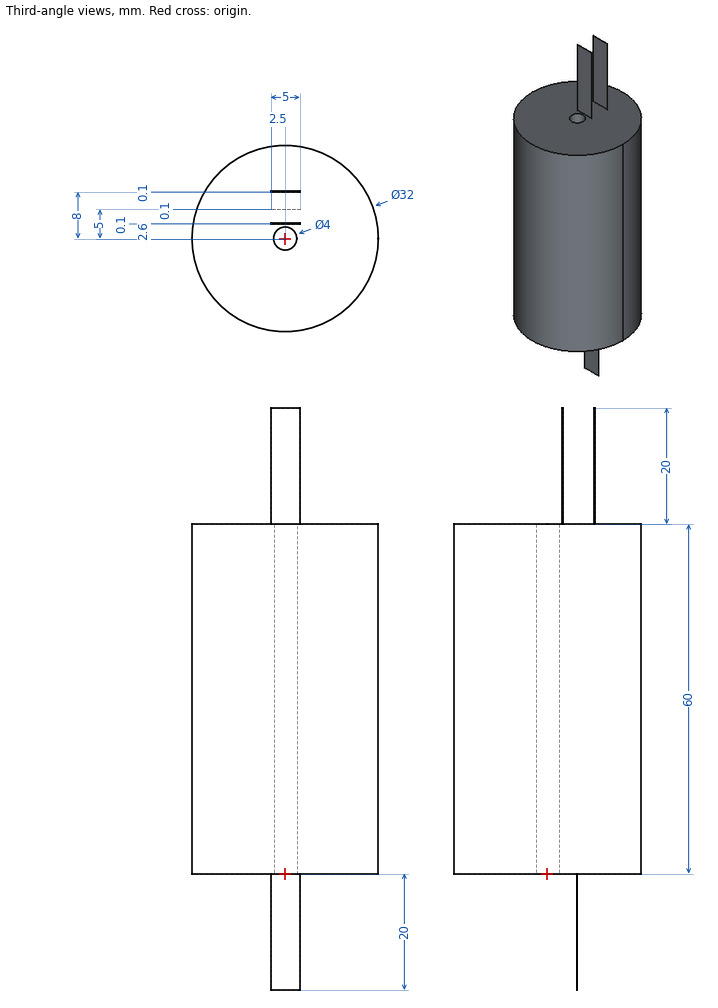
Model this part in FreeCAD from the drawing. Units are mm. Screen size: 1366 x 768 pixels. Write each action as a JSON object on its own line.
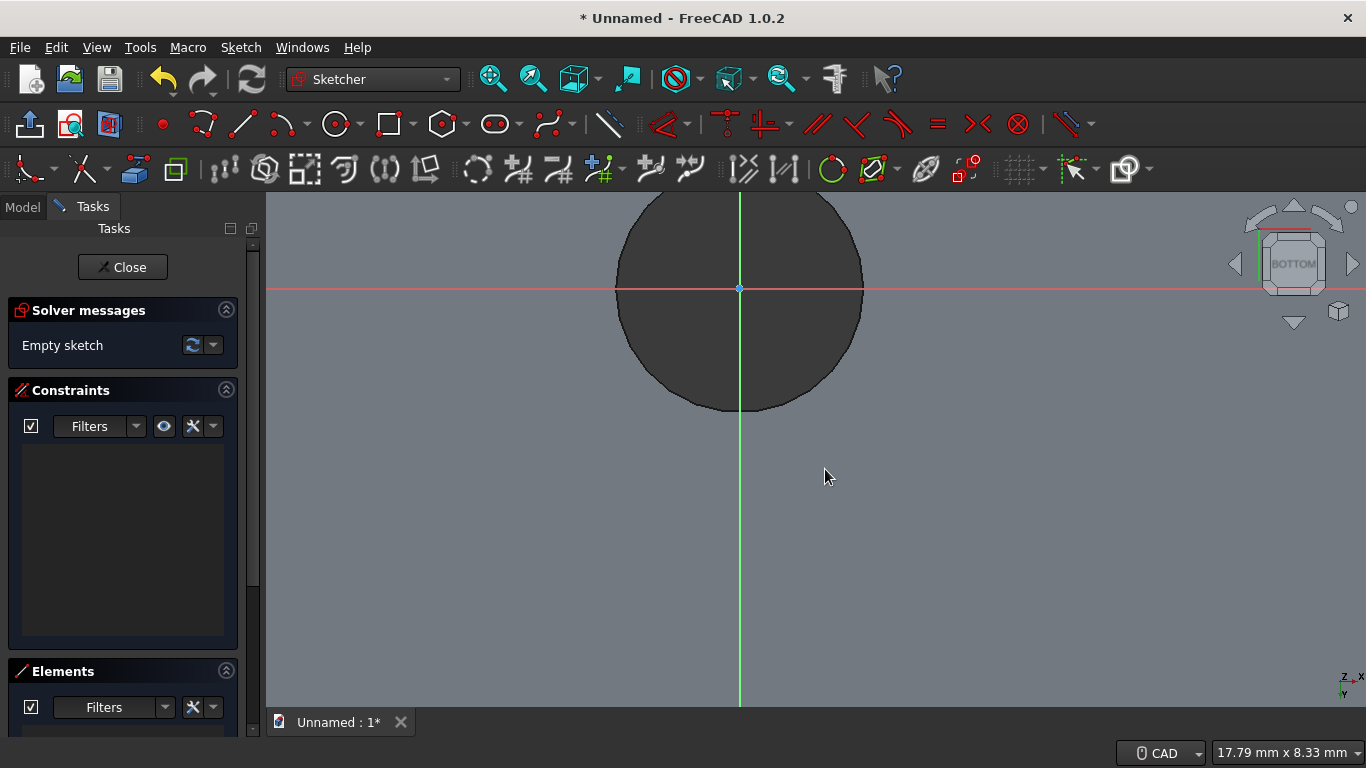
{"action": "left_click", "coordinate": [390, 124]}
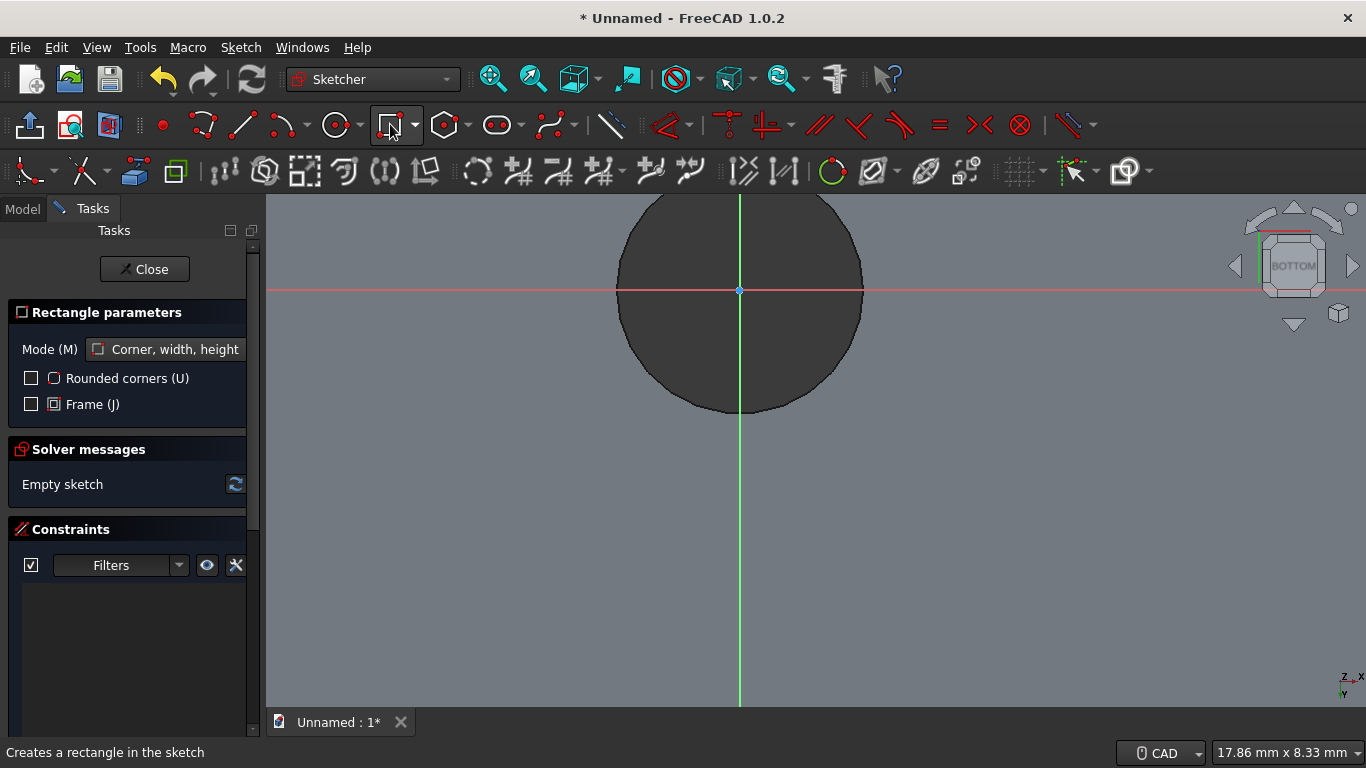
{"action": "scroll", "coordinate": [586, 598], "scroll_direction": "up", "scroll_amount": 5}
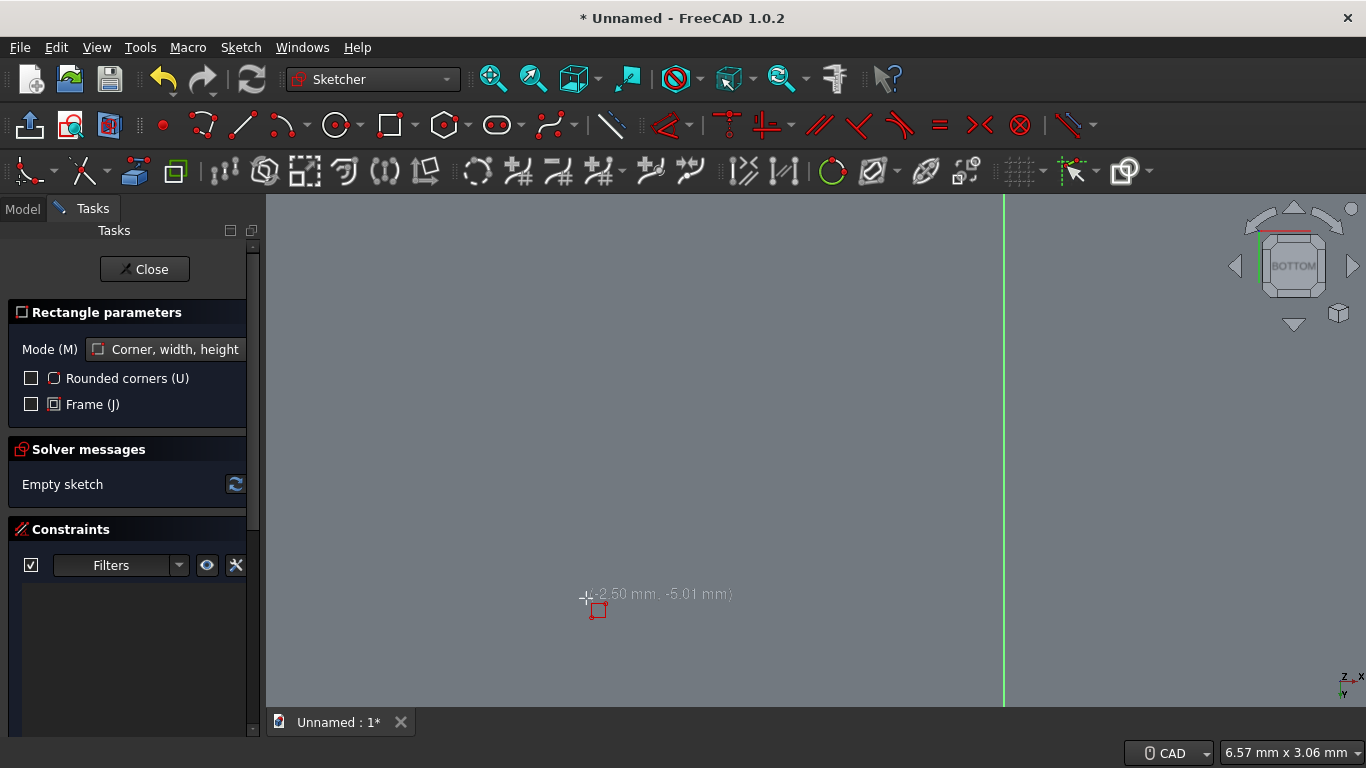
{"action": "left_click", "coordinate": [585, 598]}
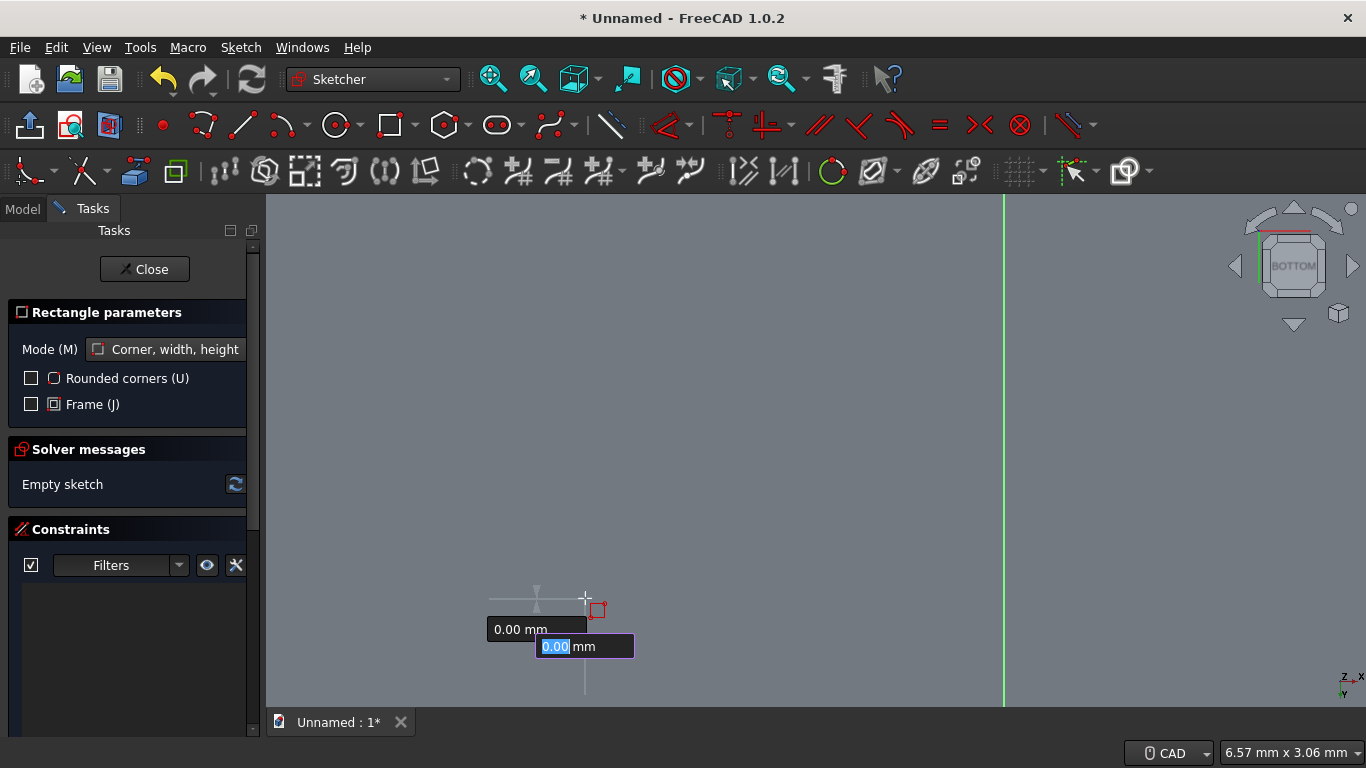
{"action": "scroll", "coordinate": [598, 604], "scroll_direction": "down", "scroll_amount": 5}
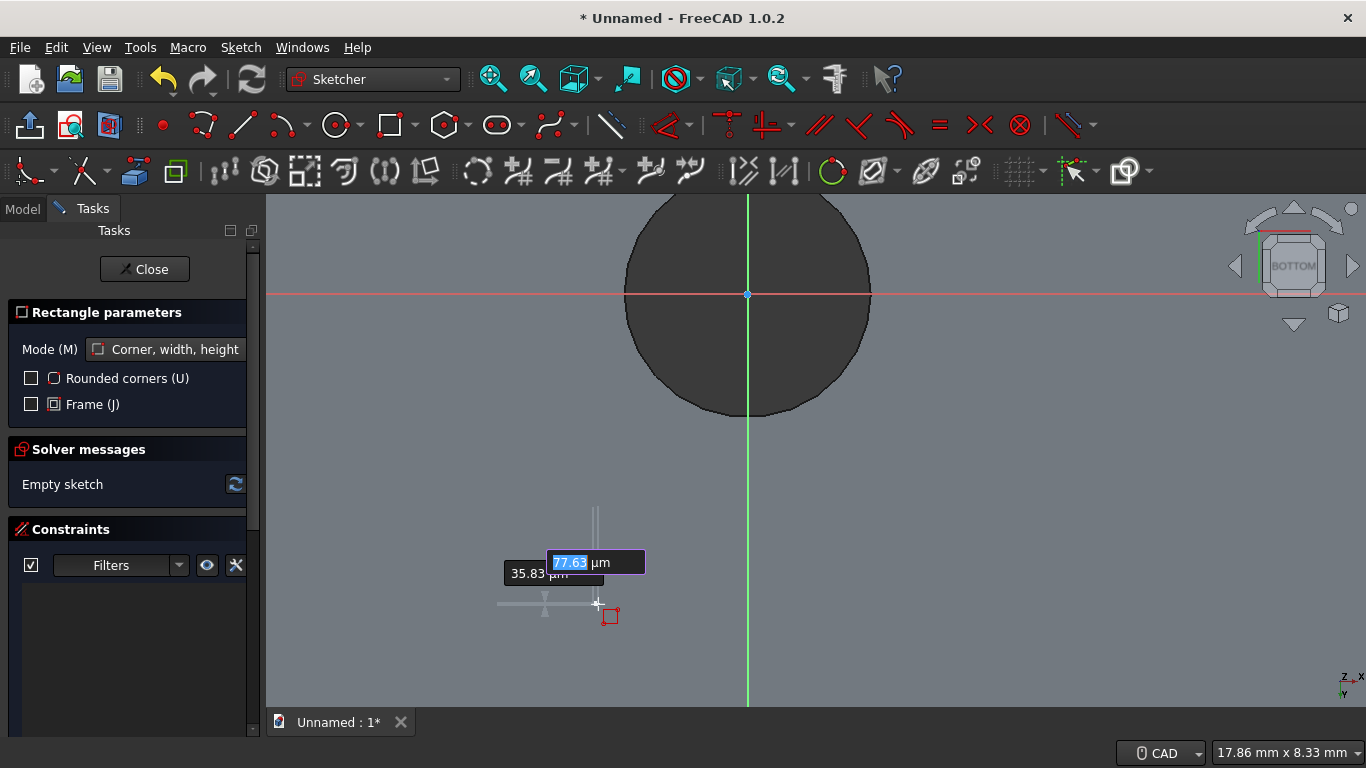
{"action": "left_click", "coordinate": [902, 608]}
{"action": "key", "text": "Escape"}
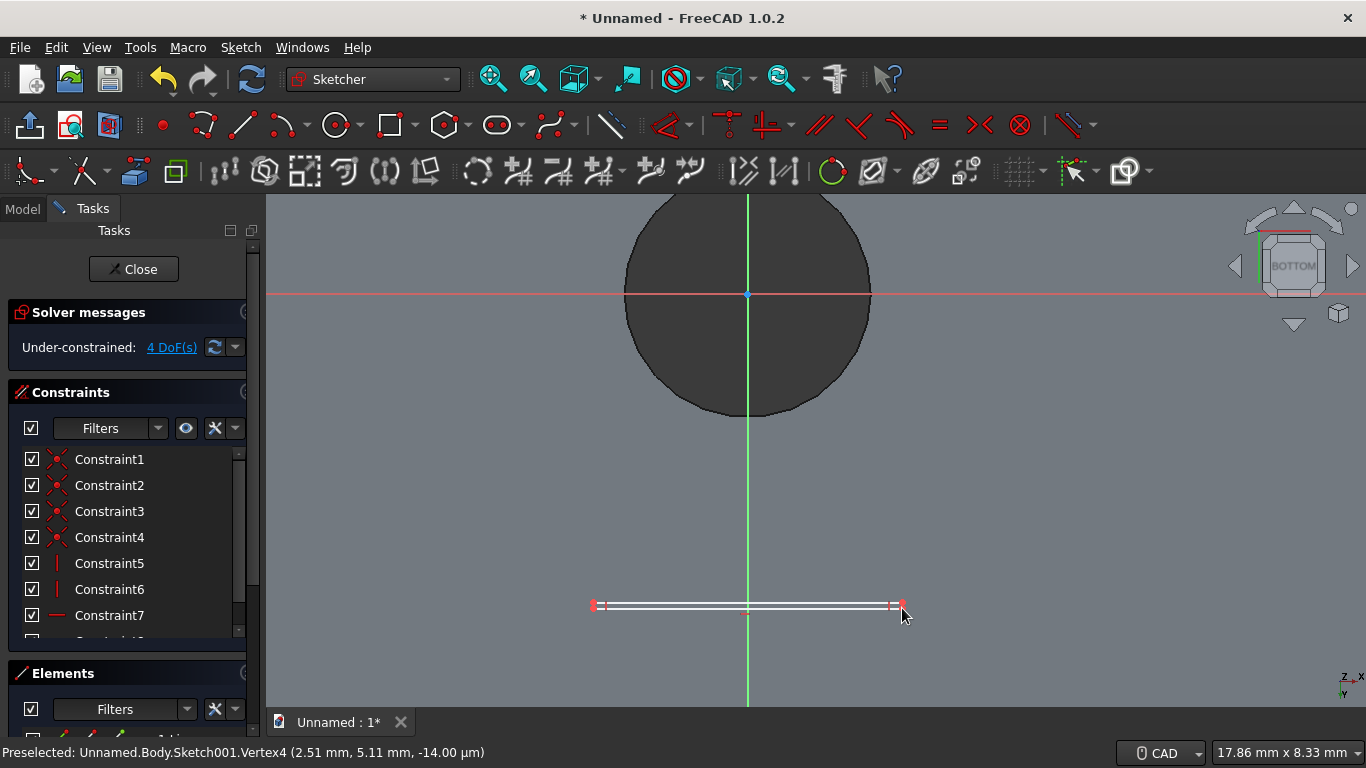
{"action": "scroll", "coordinate": [686, 609], "scroll_direction": "up", "scroll_amount": 4}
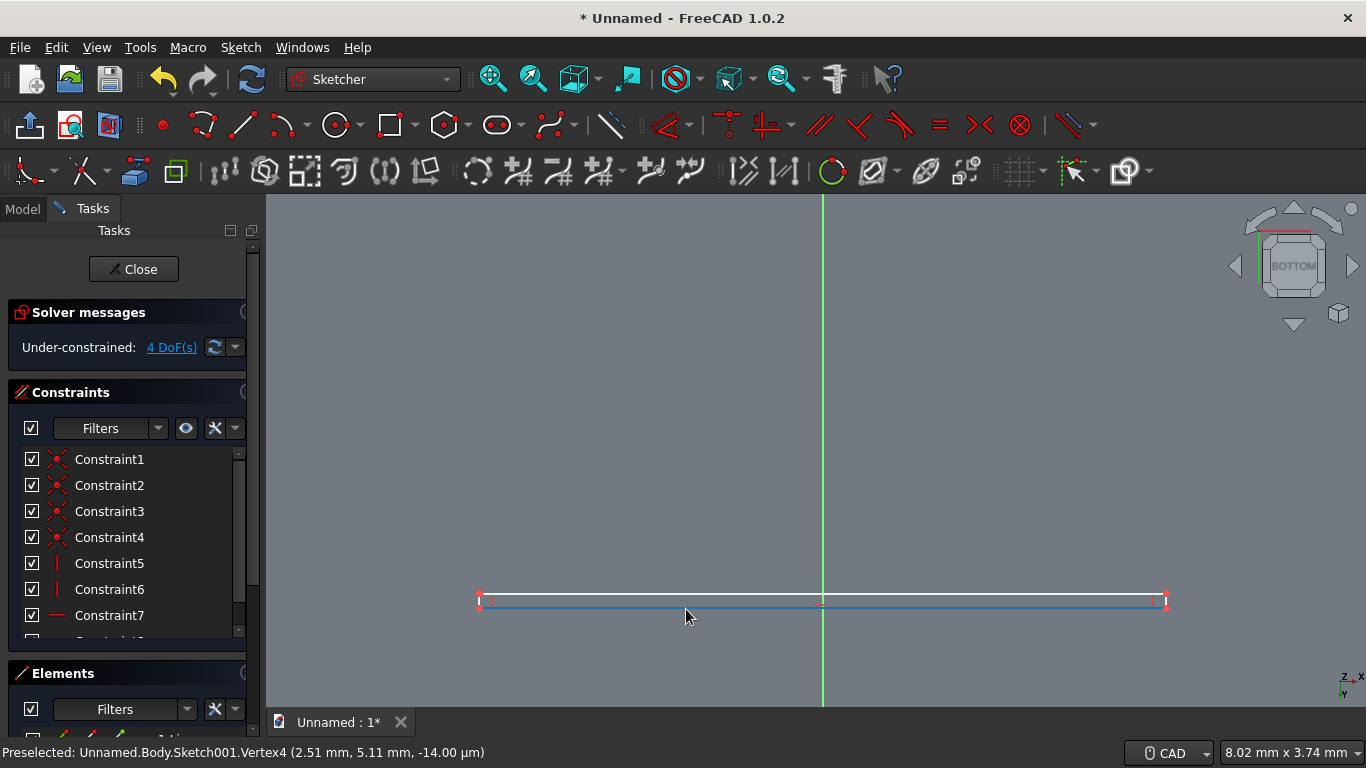
{"action": "left_click", "coordinate": [686, 608]}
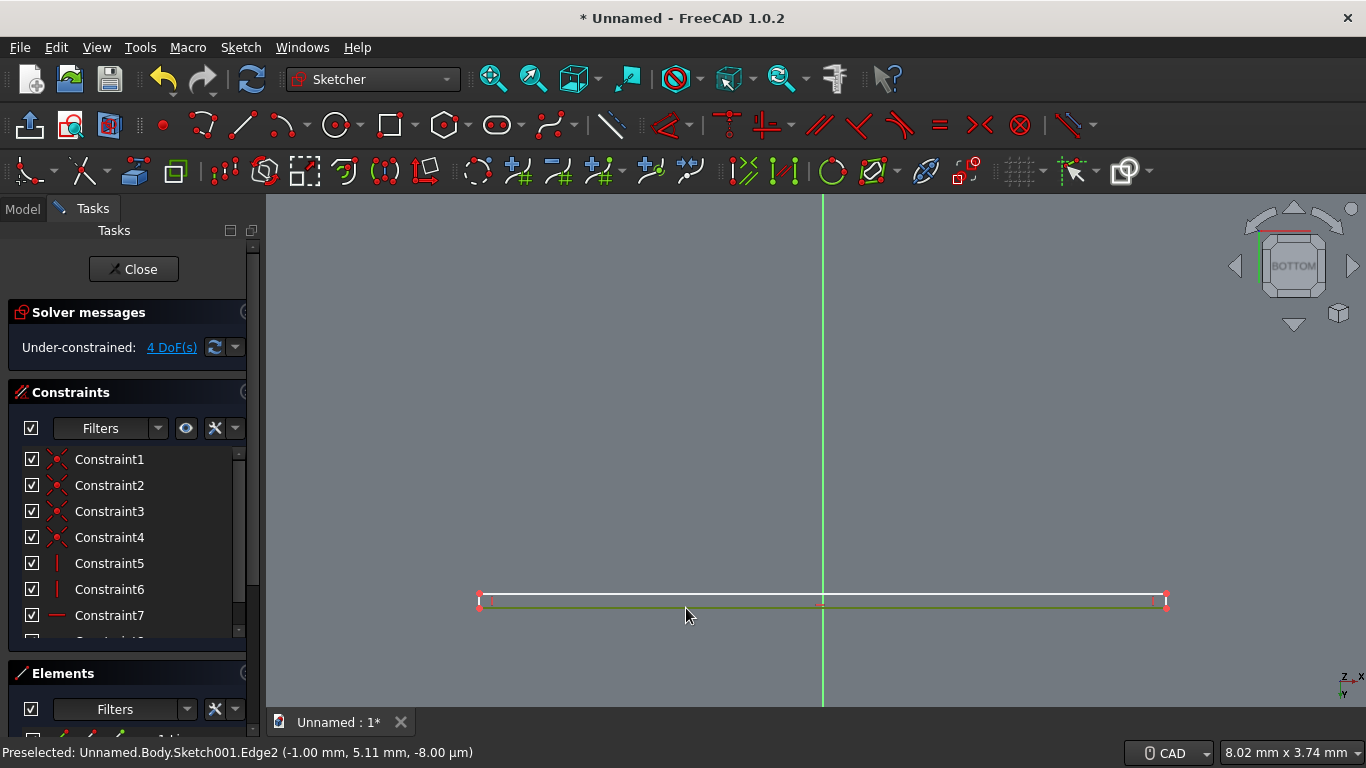
{"action": "left_click", "coordinate": [692, 126]}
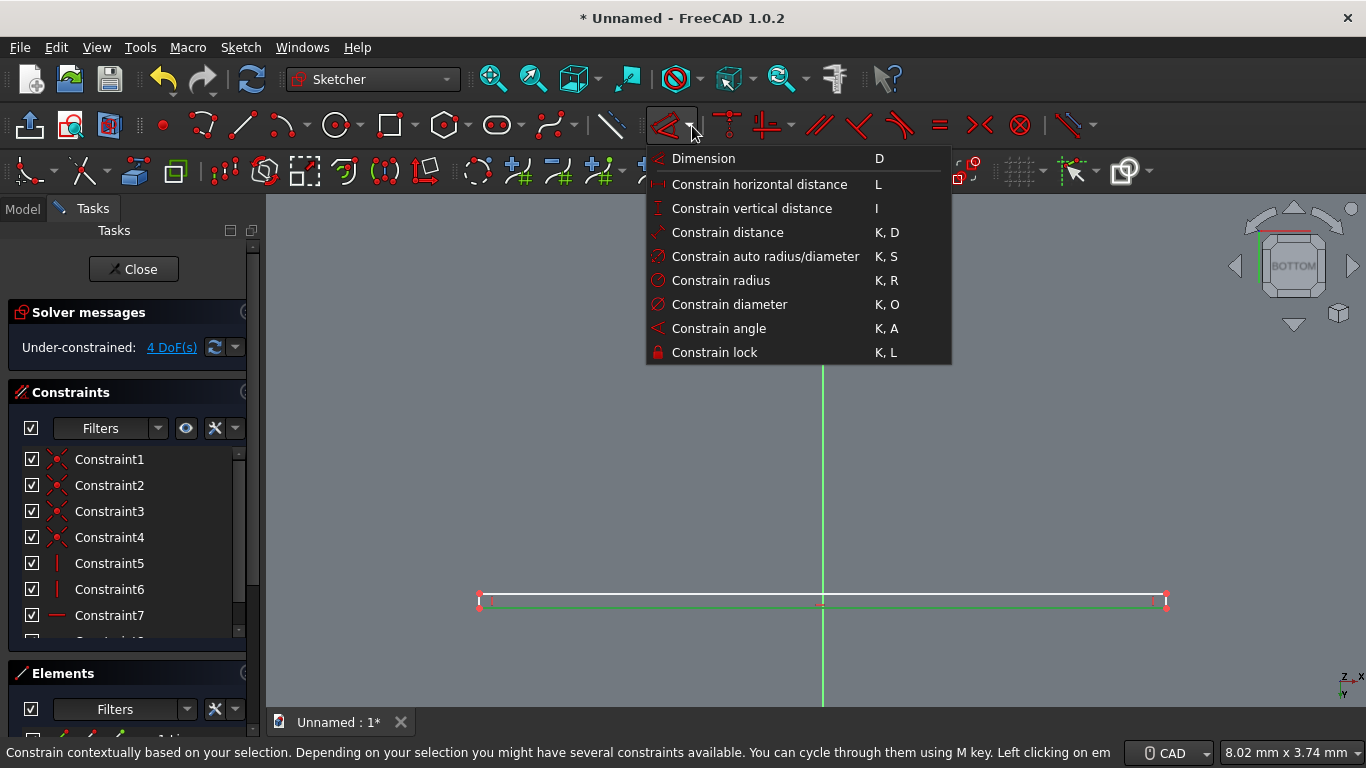
{"action": "left_click", "coordinate": [799, 184]}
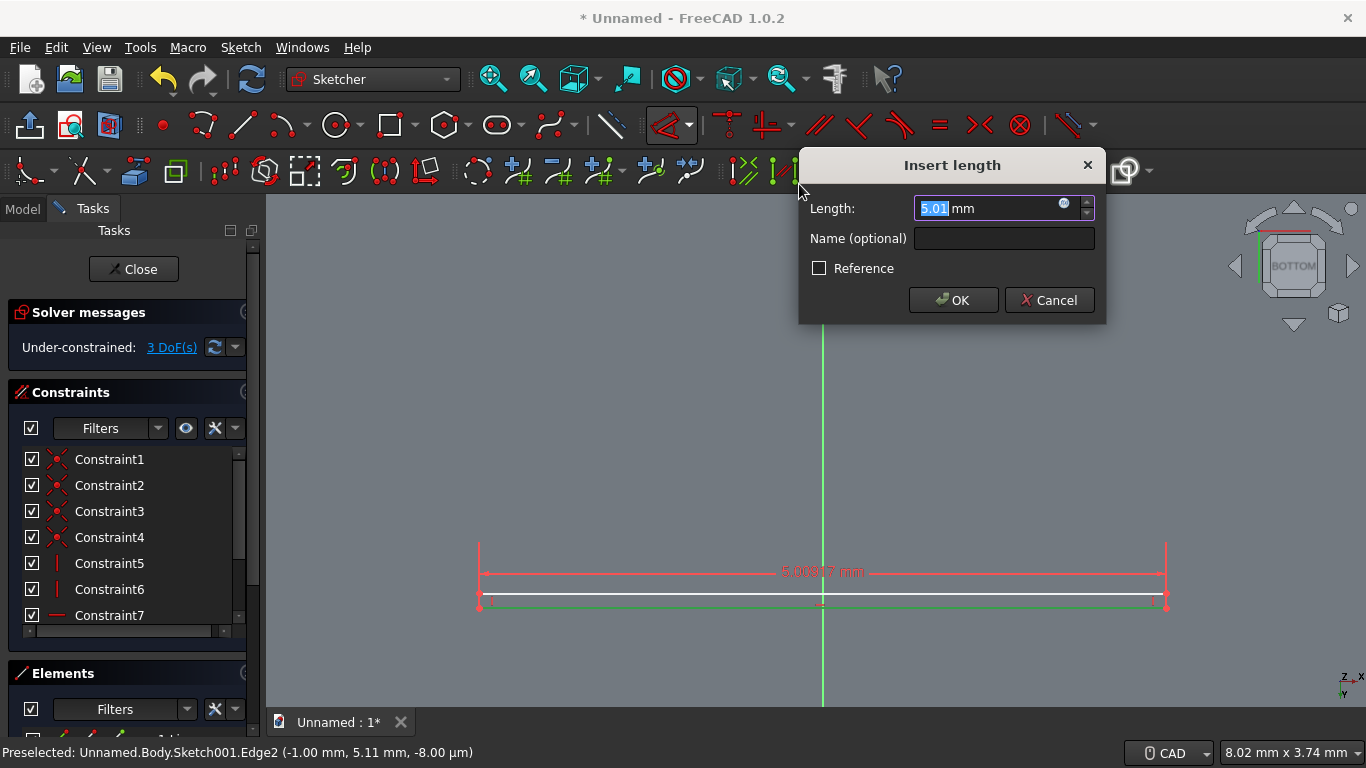
{"action": "type", "text": "5"}
{"action": "key", "text": "Return"}